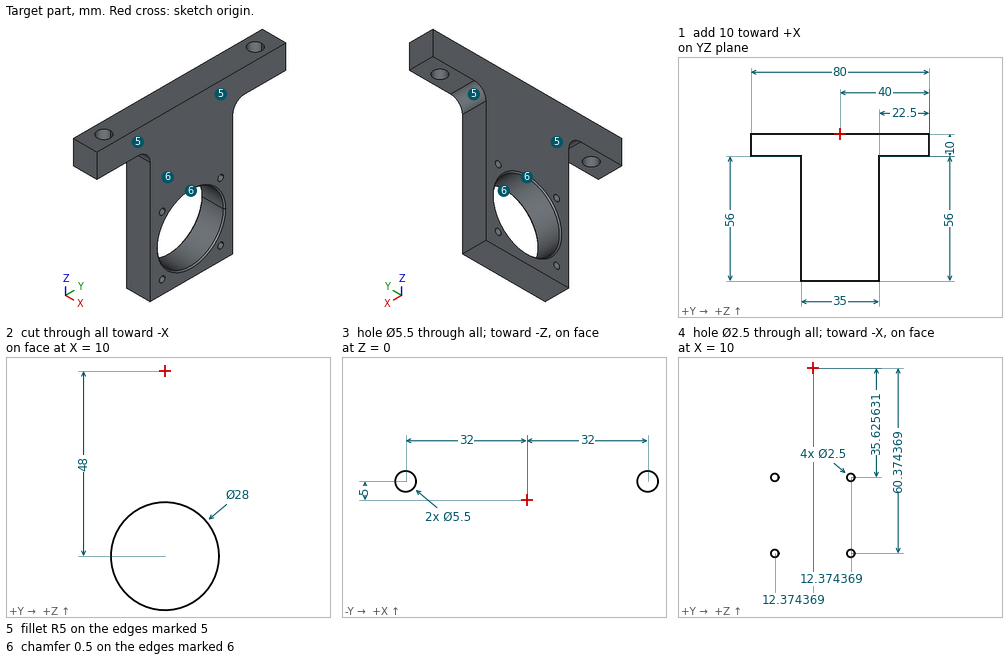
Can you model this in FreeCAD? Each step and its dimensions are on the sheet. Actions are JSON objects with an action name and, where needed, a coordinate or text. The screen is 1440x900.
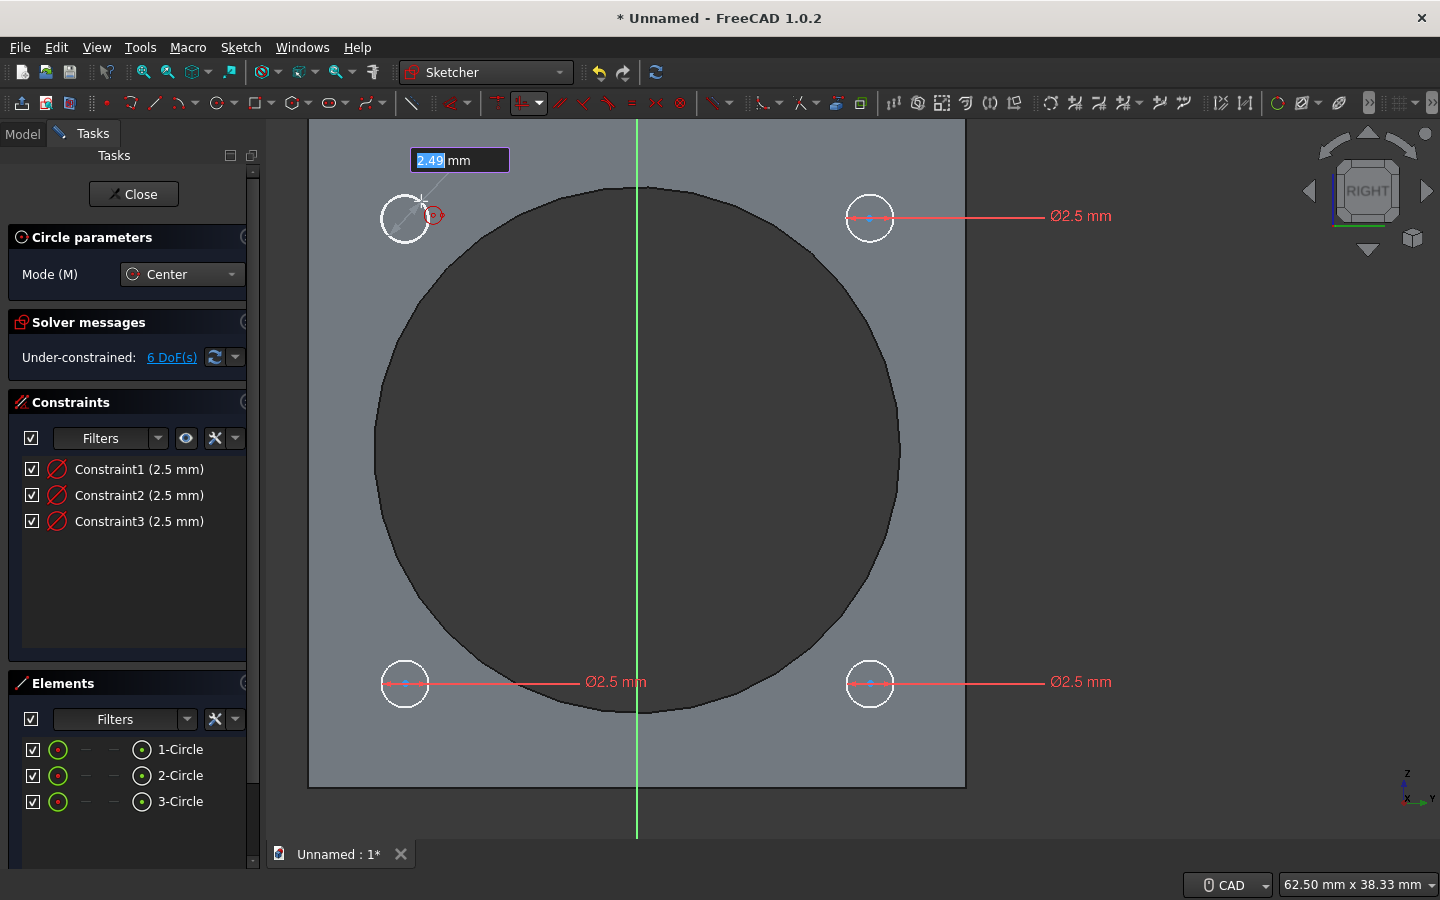
{"action": "type", "text": "2.5"}
{"action": "key", "text": "Return"}
{"action": "key", "text": "Escape"}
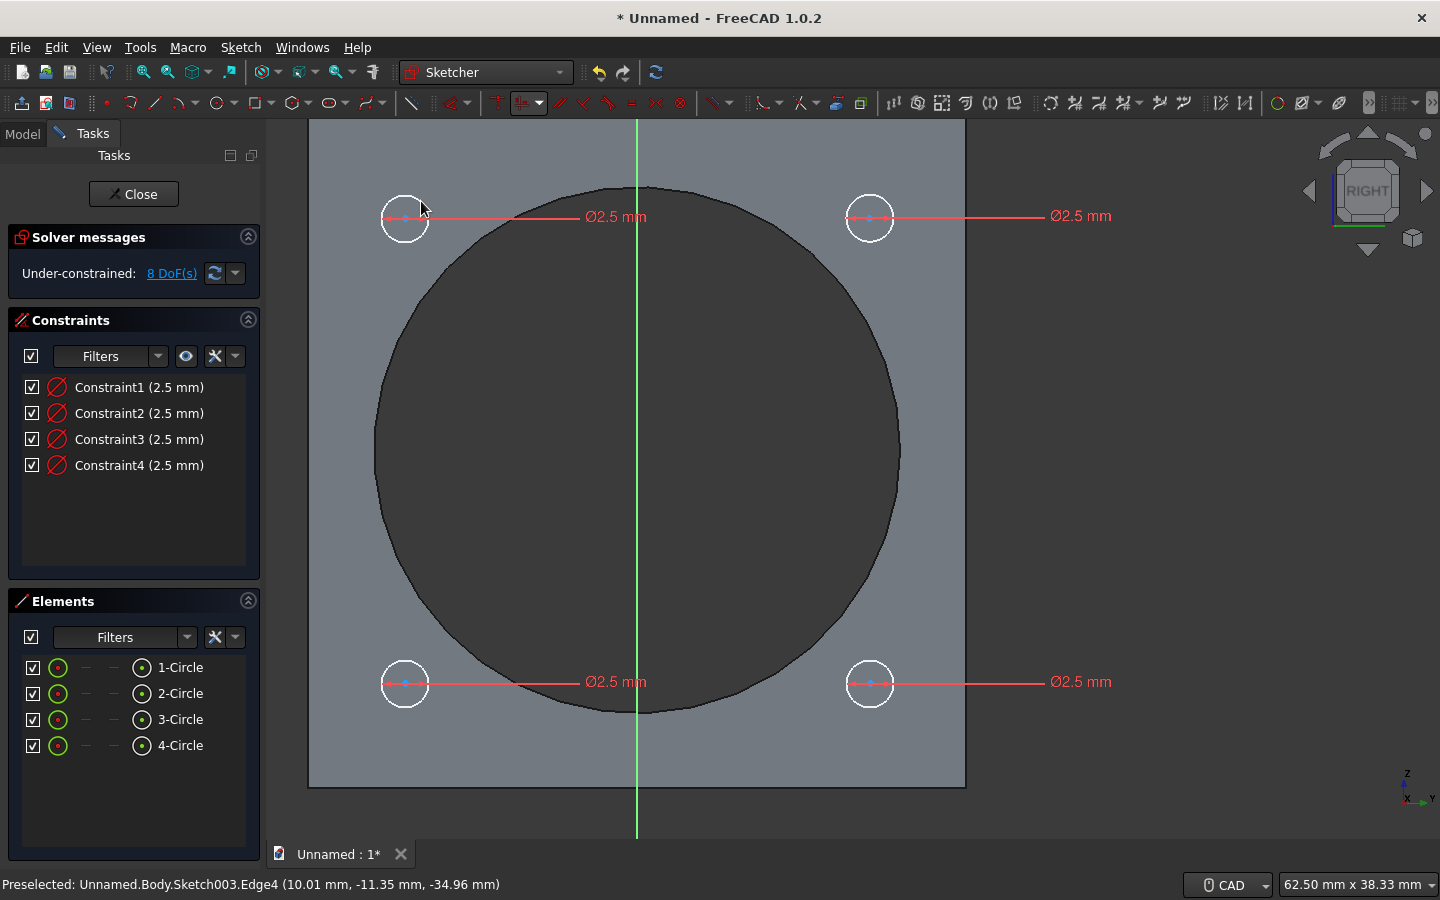
{"action": "left_click", "coordinate": [870, 218]}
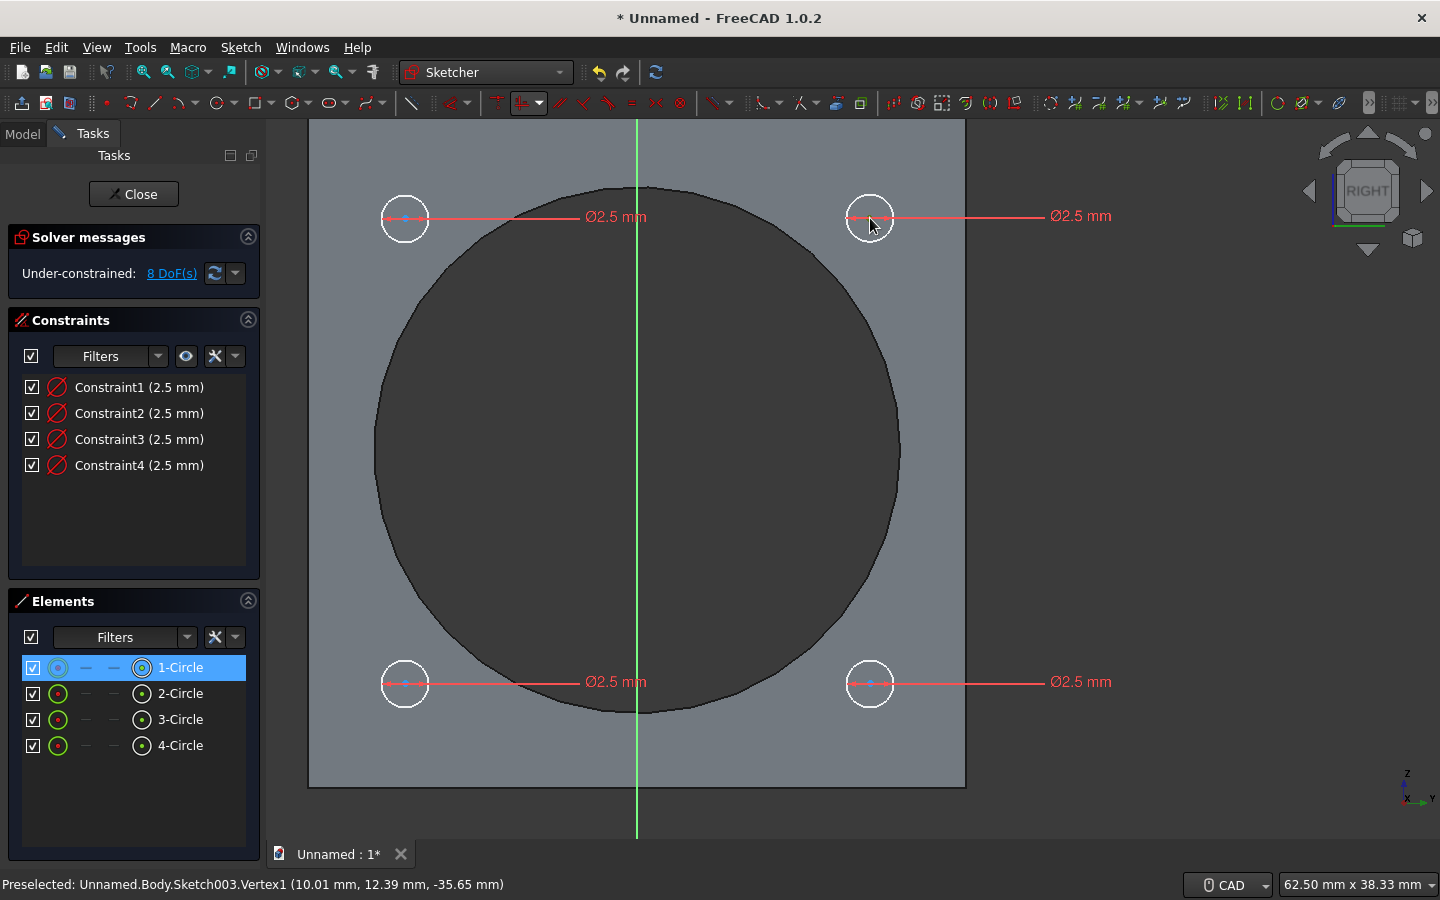
{"action": "left_click", "coordinate": [870, 684]}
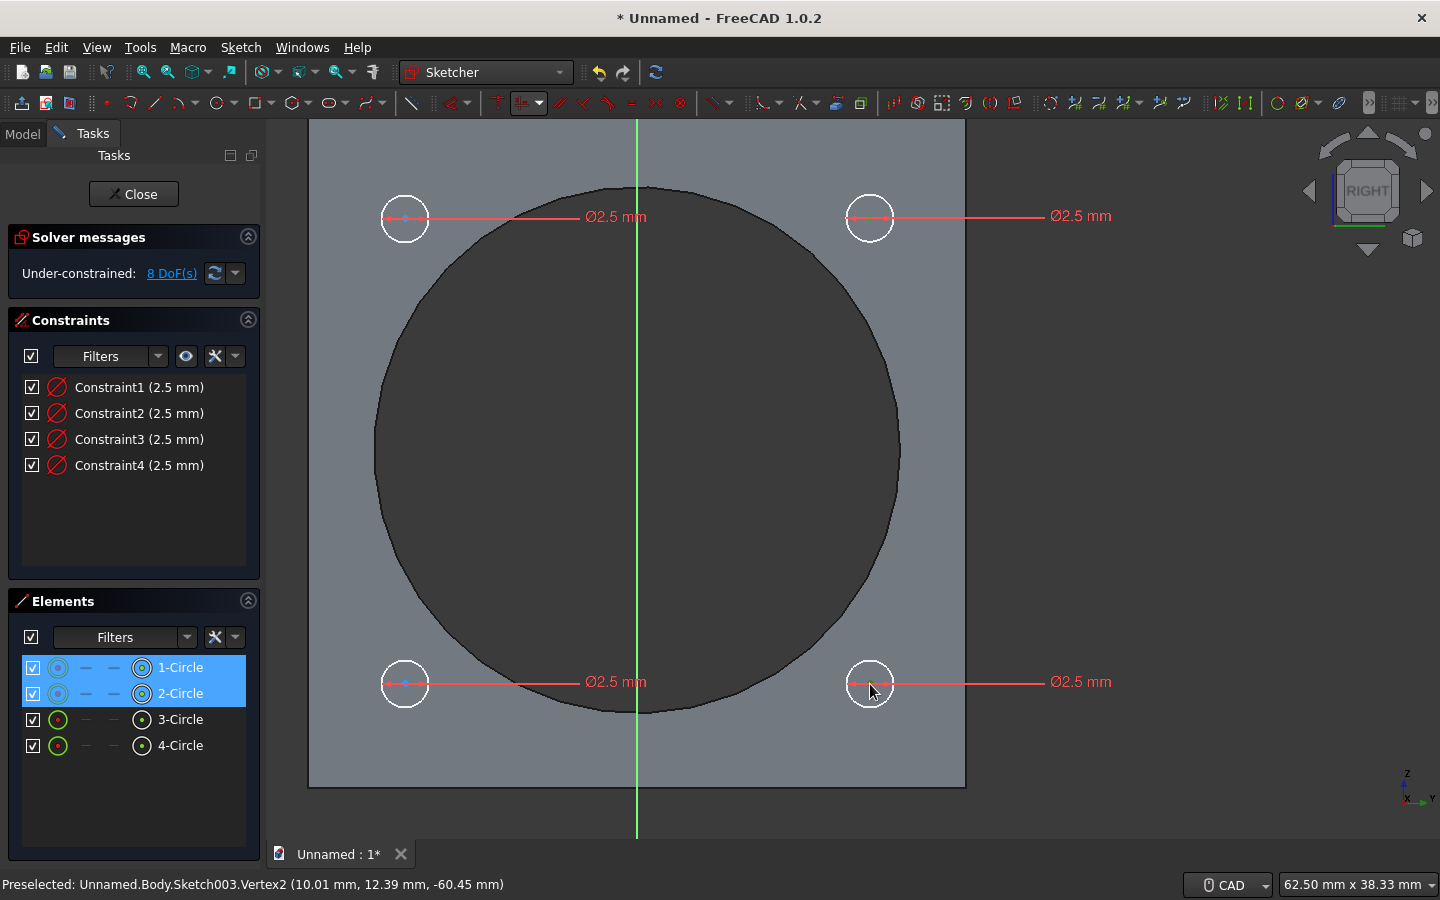
{"action": "key", "text": "v"}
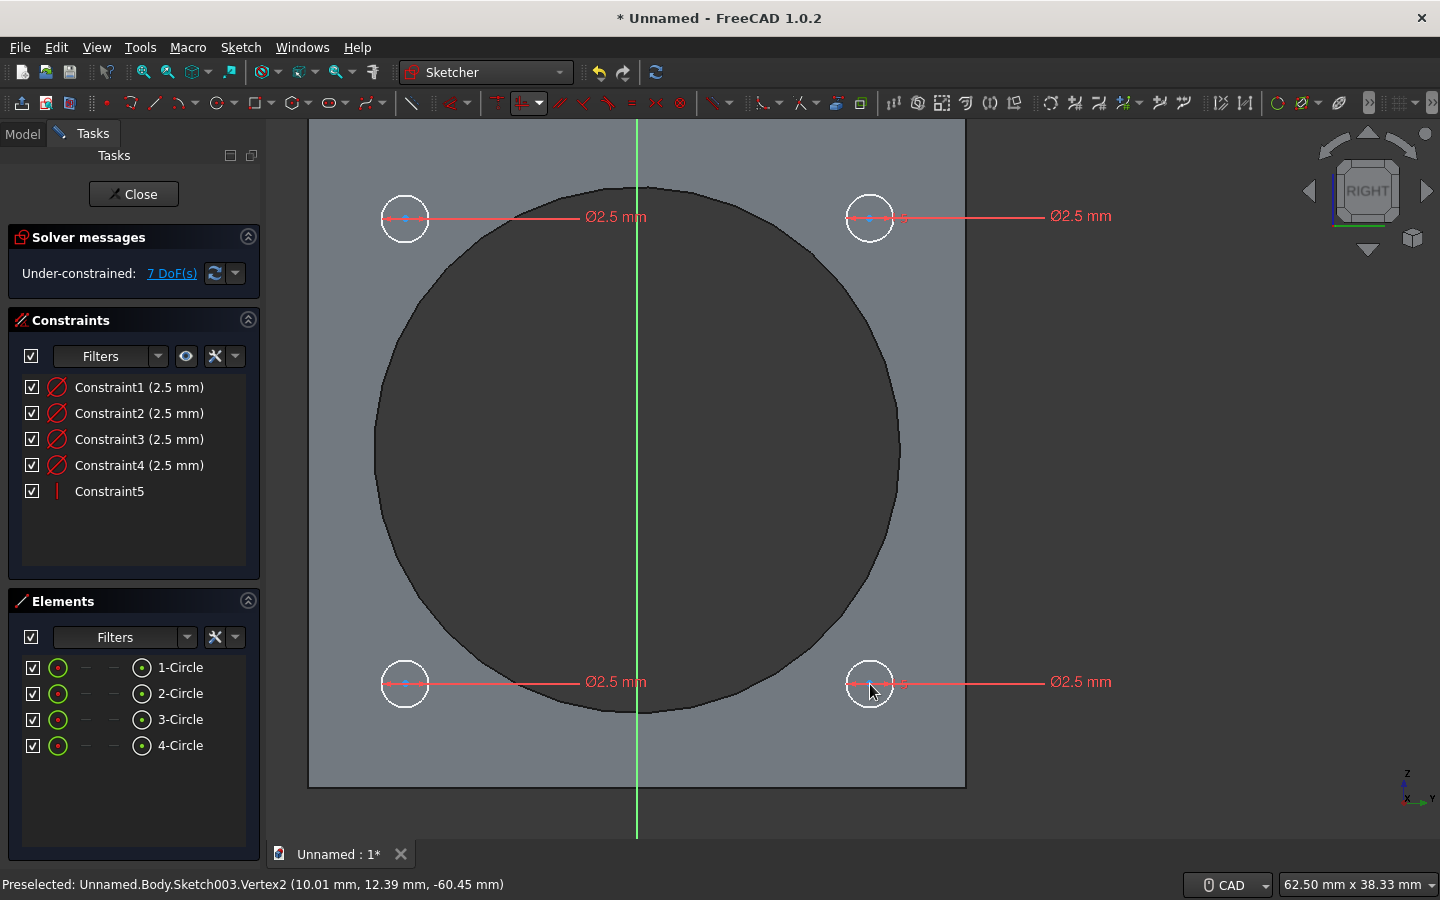
{"action": "left_click", "coordinate": [870, 684]}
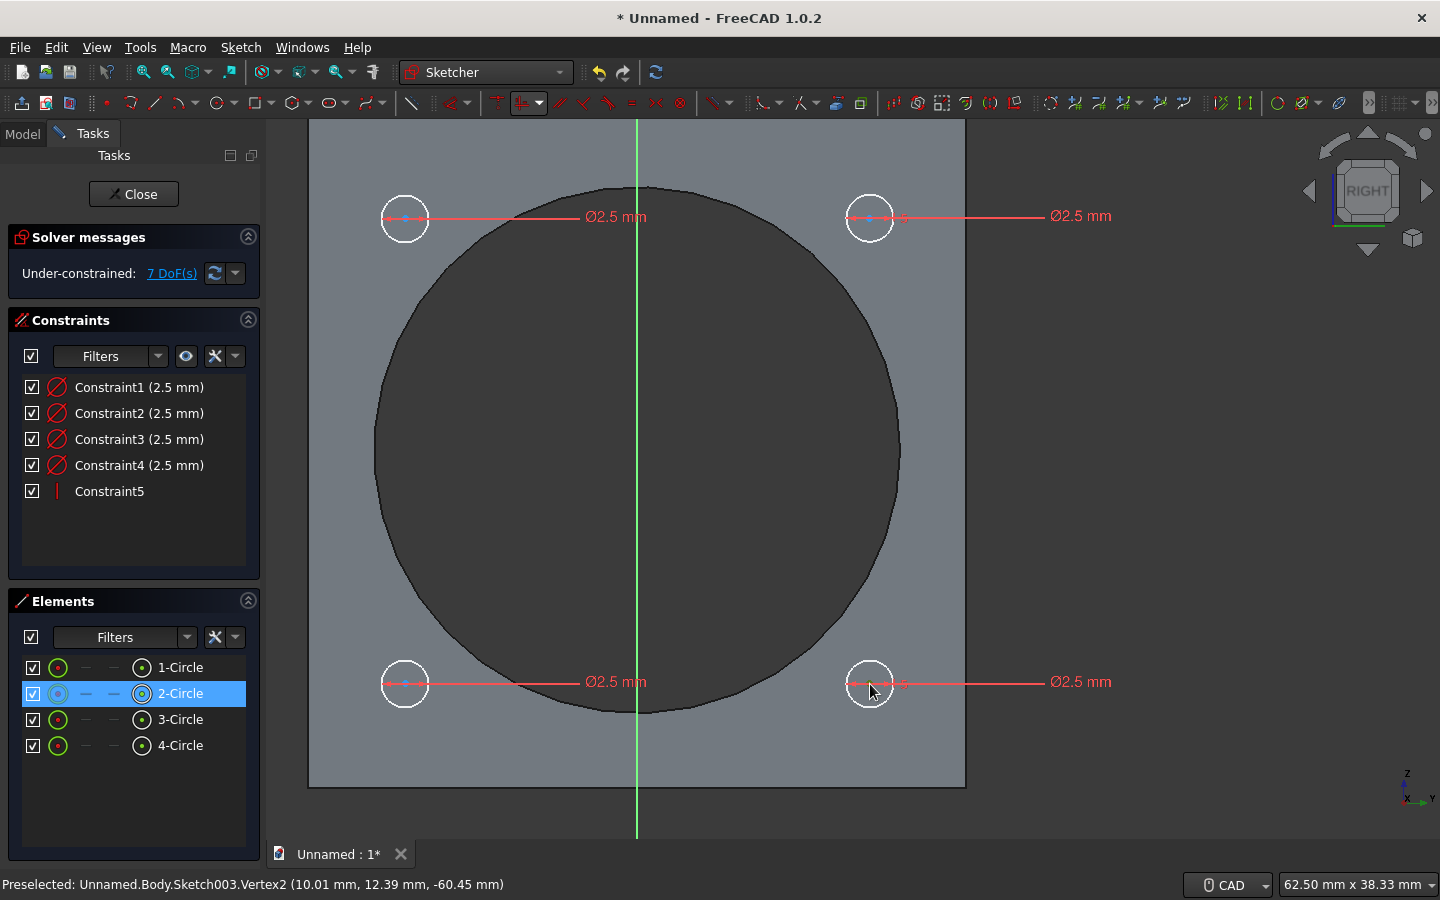
{"action": "left_click", "coordinate": [405, 684]}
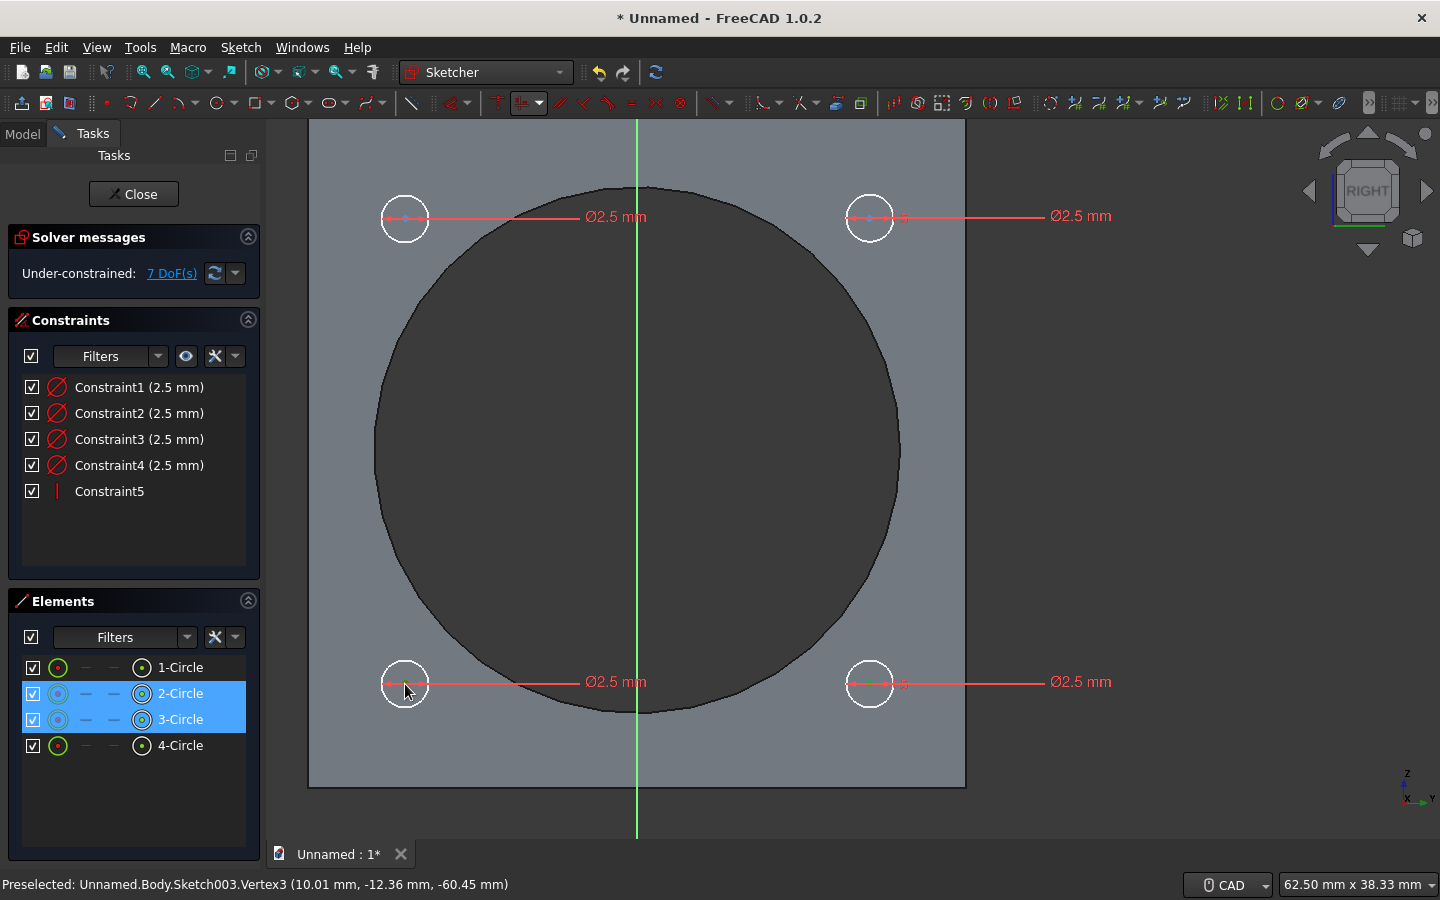
{"action": "left_click", "coordinate": [542, 104]}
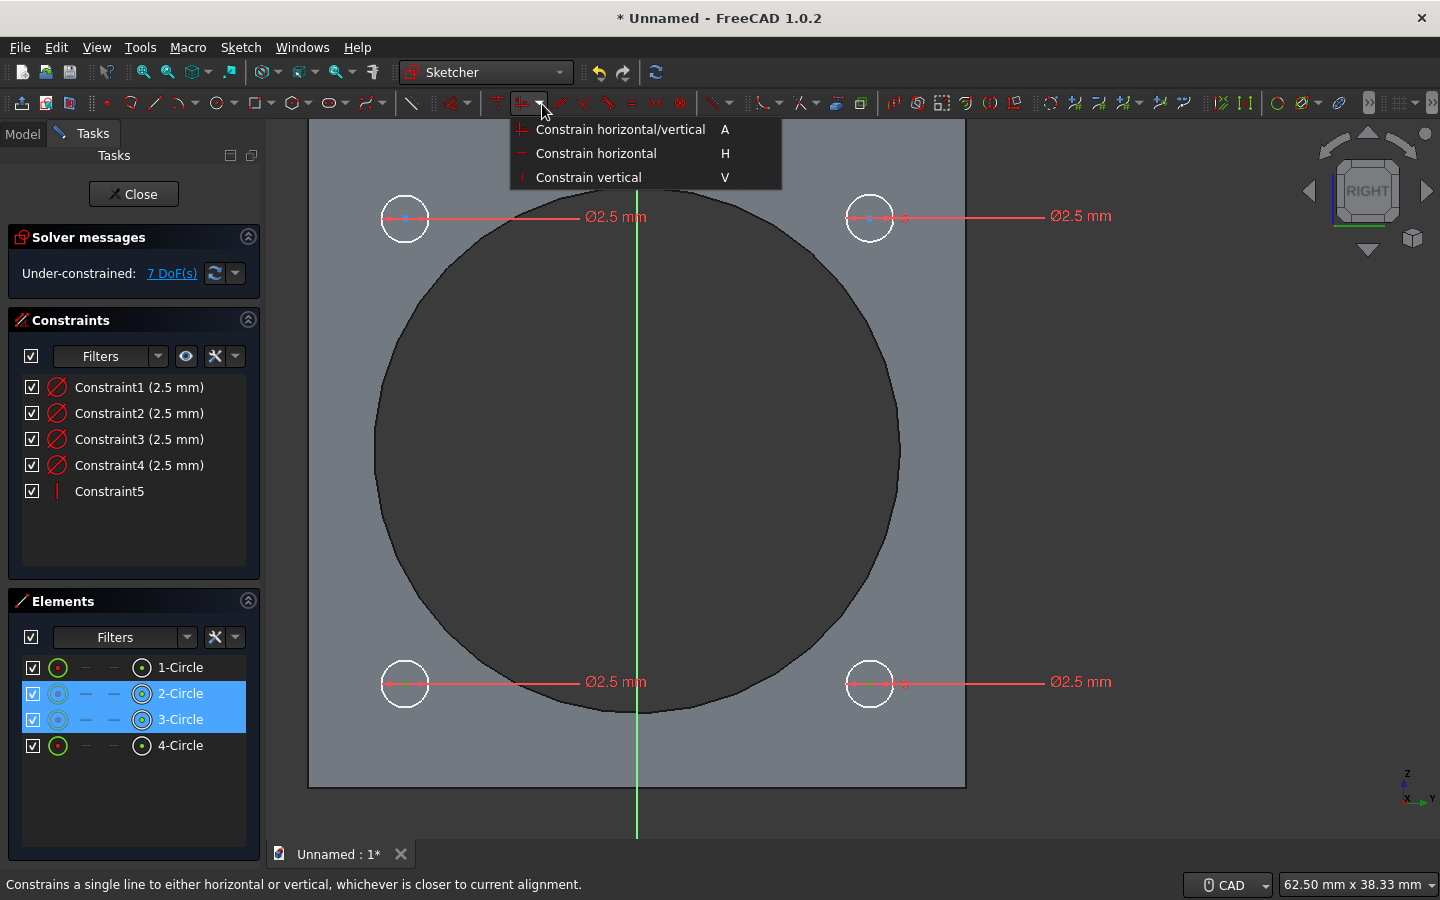
{"action": "left_click", "coordinate": [646, 153]}